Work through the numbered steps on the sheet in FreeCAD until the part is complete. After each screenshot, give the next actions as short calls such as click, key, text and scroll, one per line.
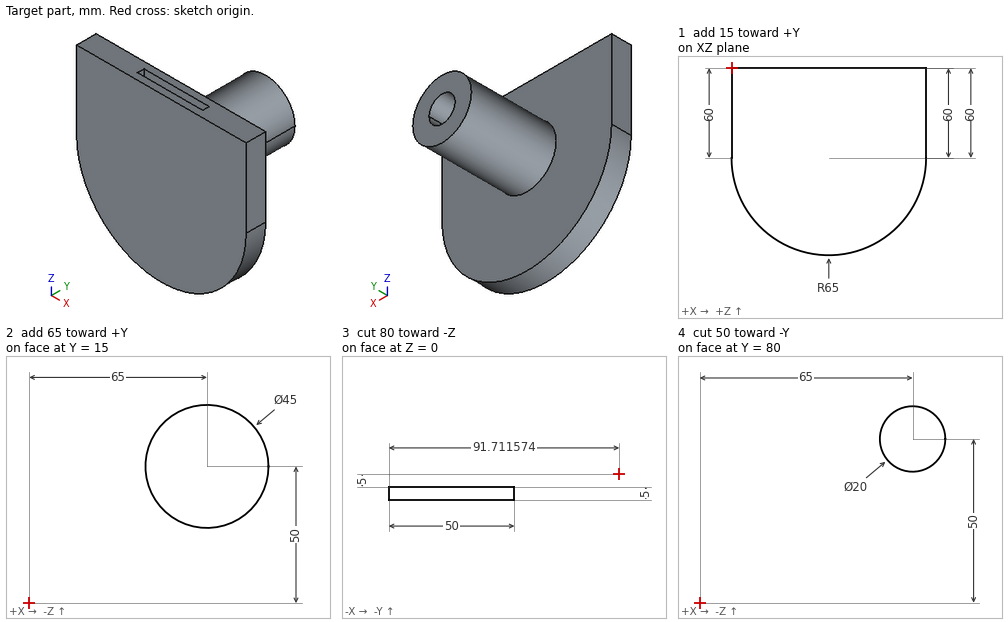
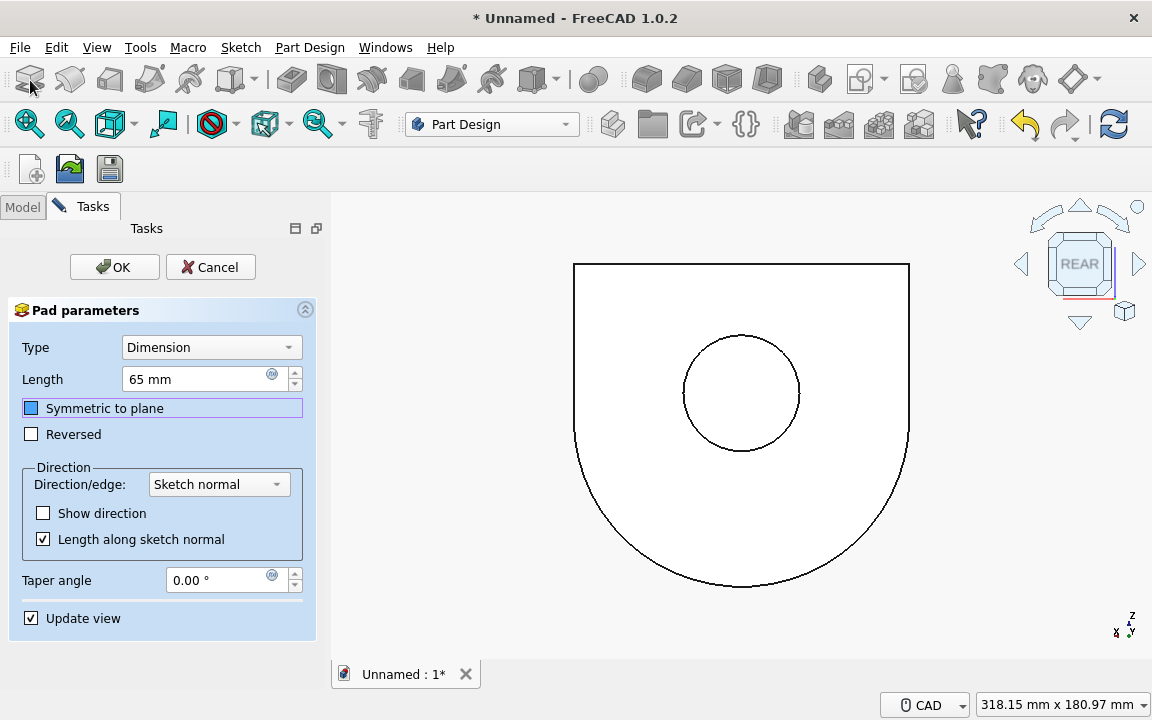
click(115, 267)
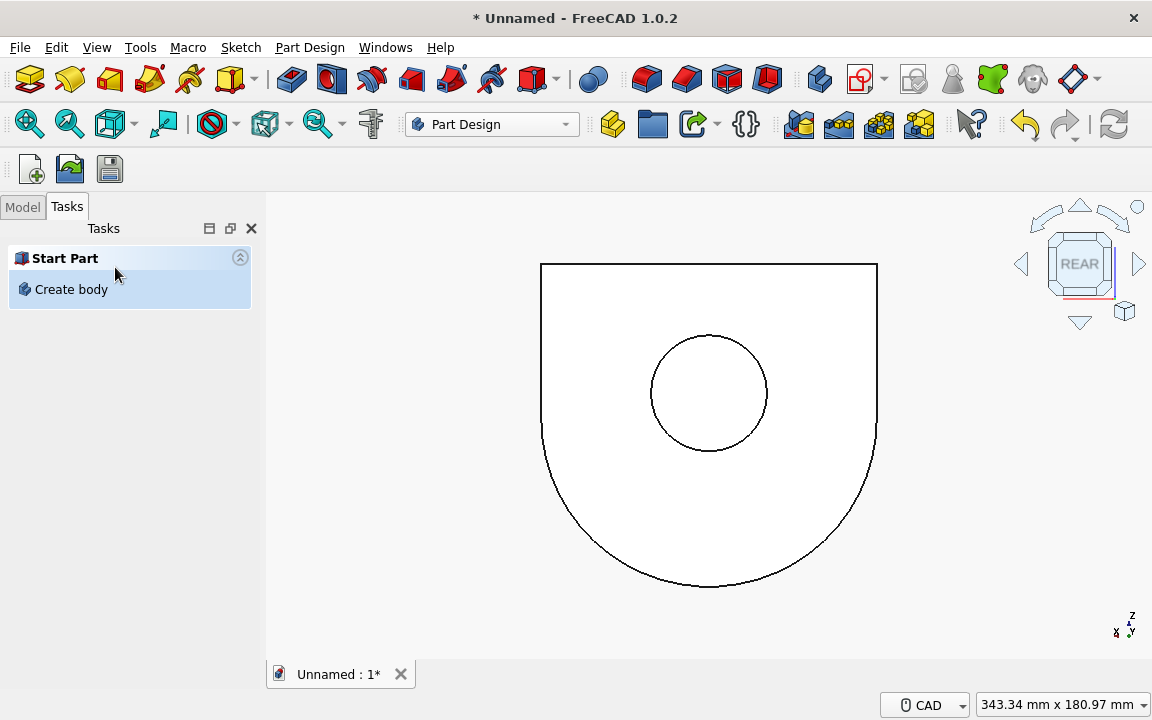
key(0)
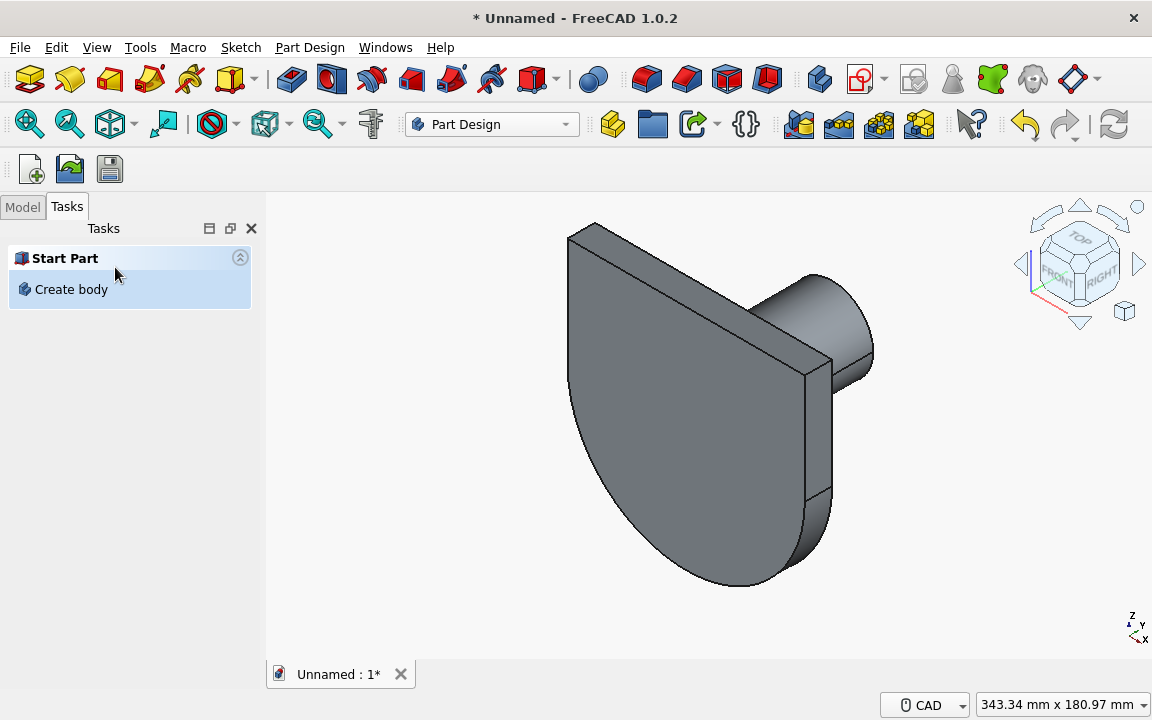
click(30, 124)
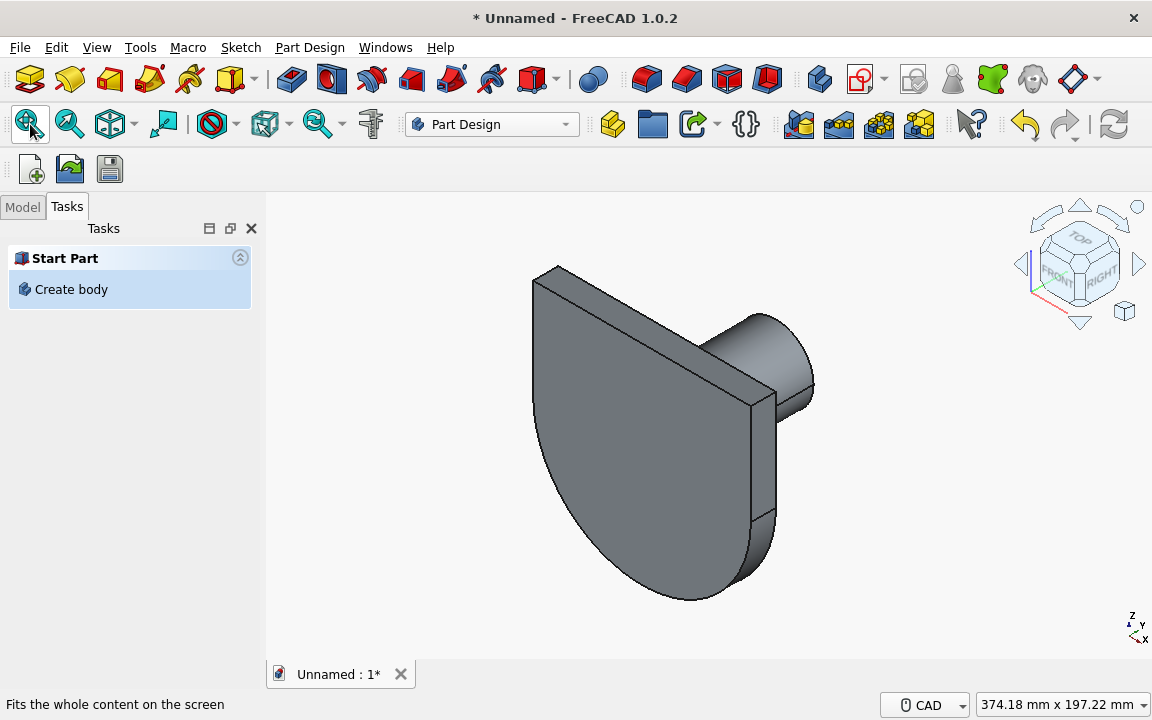
click(748, 389)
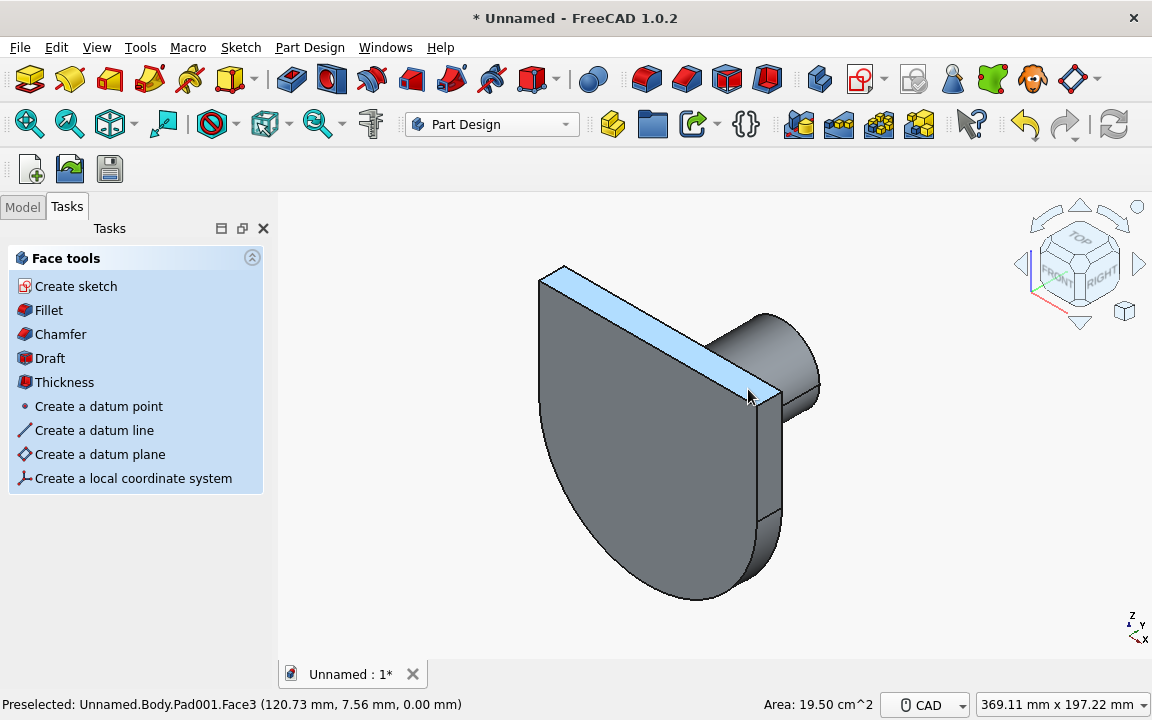
click(860, 80)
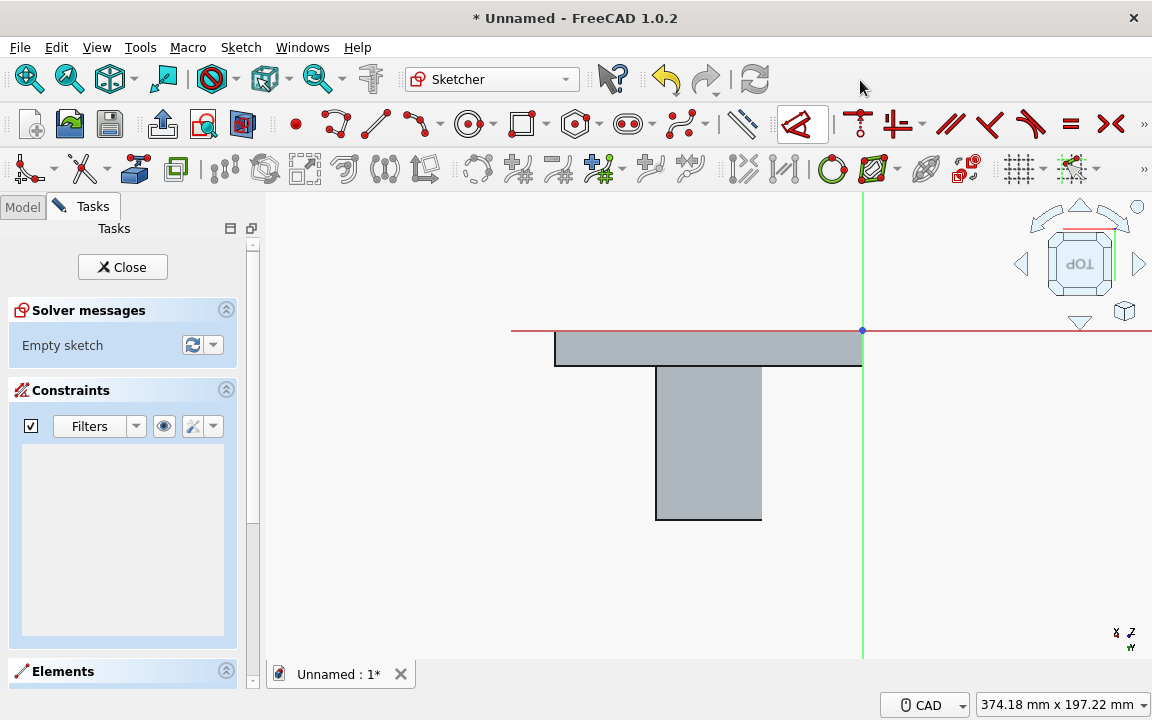
scroll(847, 275, up, 4)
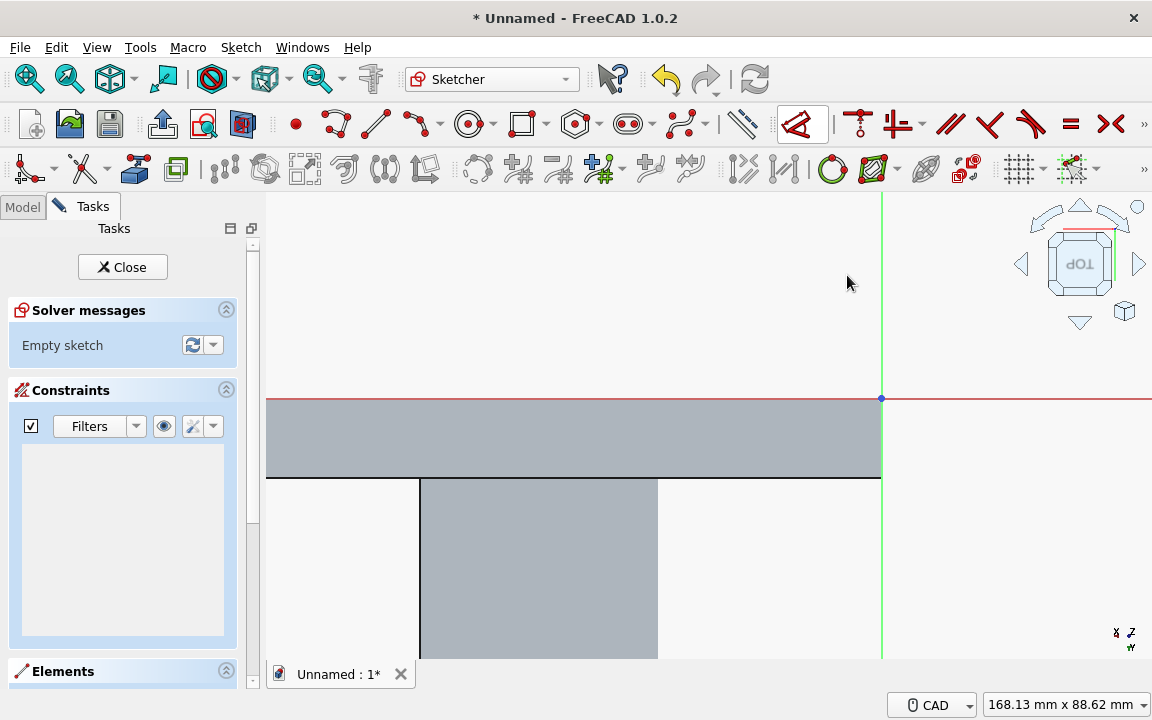
click(522, 124)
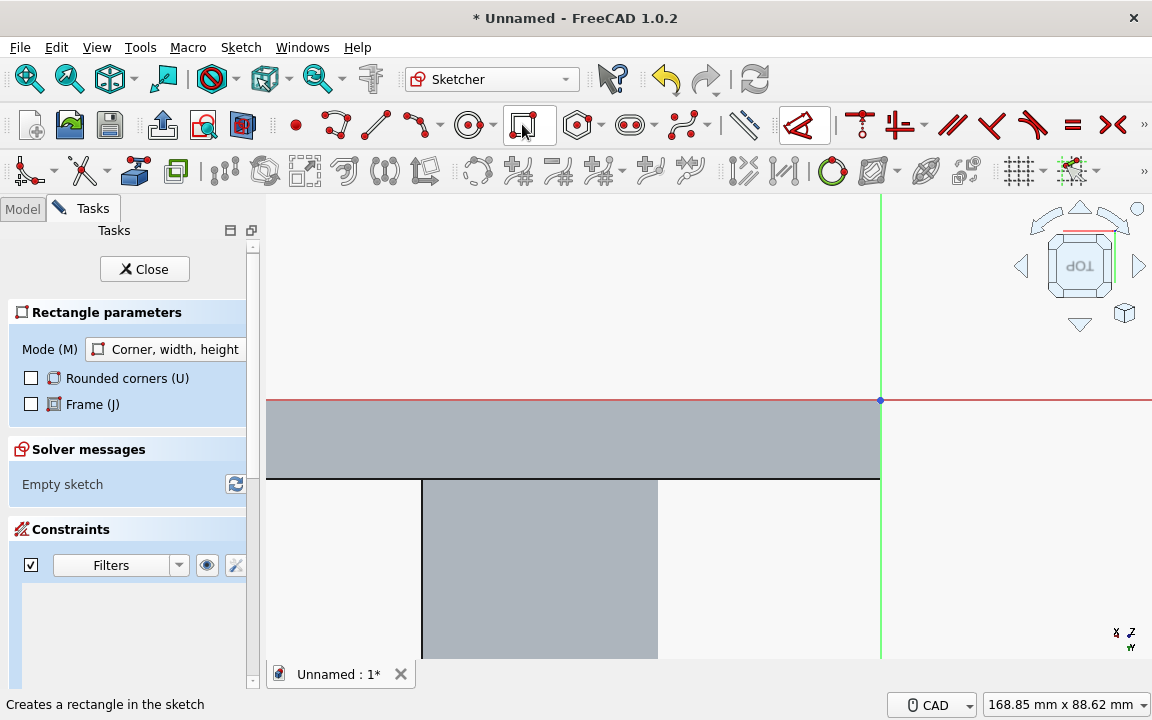
click(400, 426)
move(662, 453)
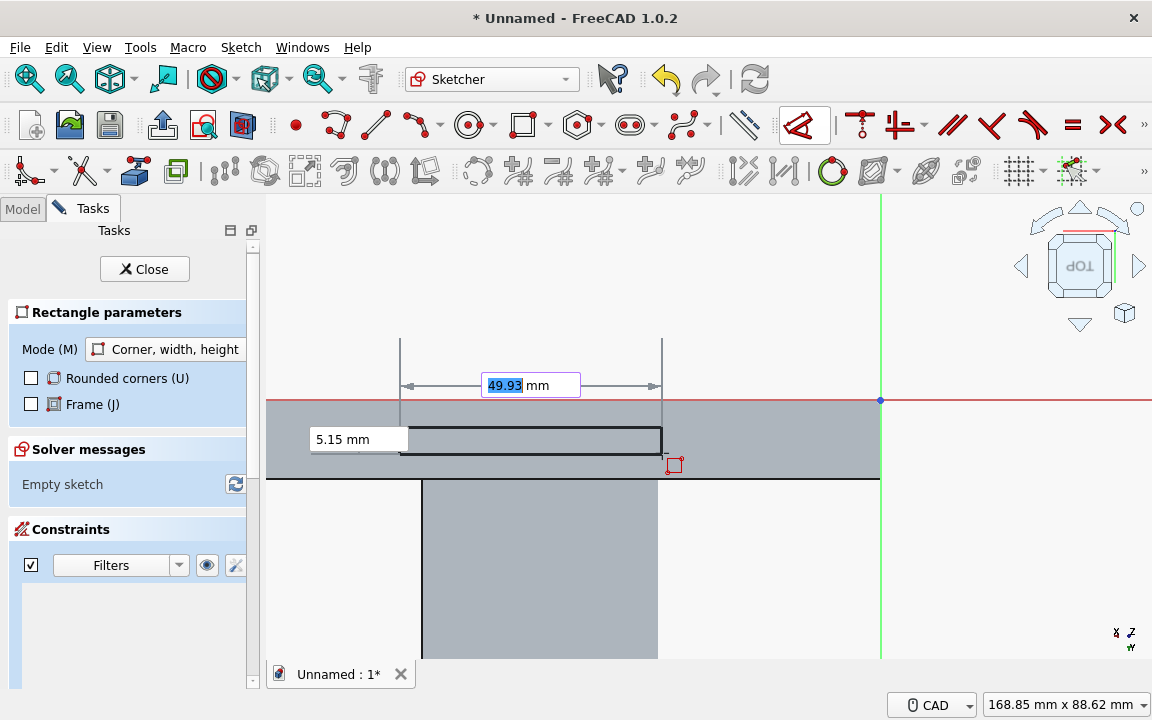
text(50)
key(Tab)
text(5)
key(Return)
key(Escape)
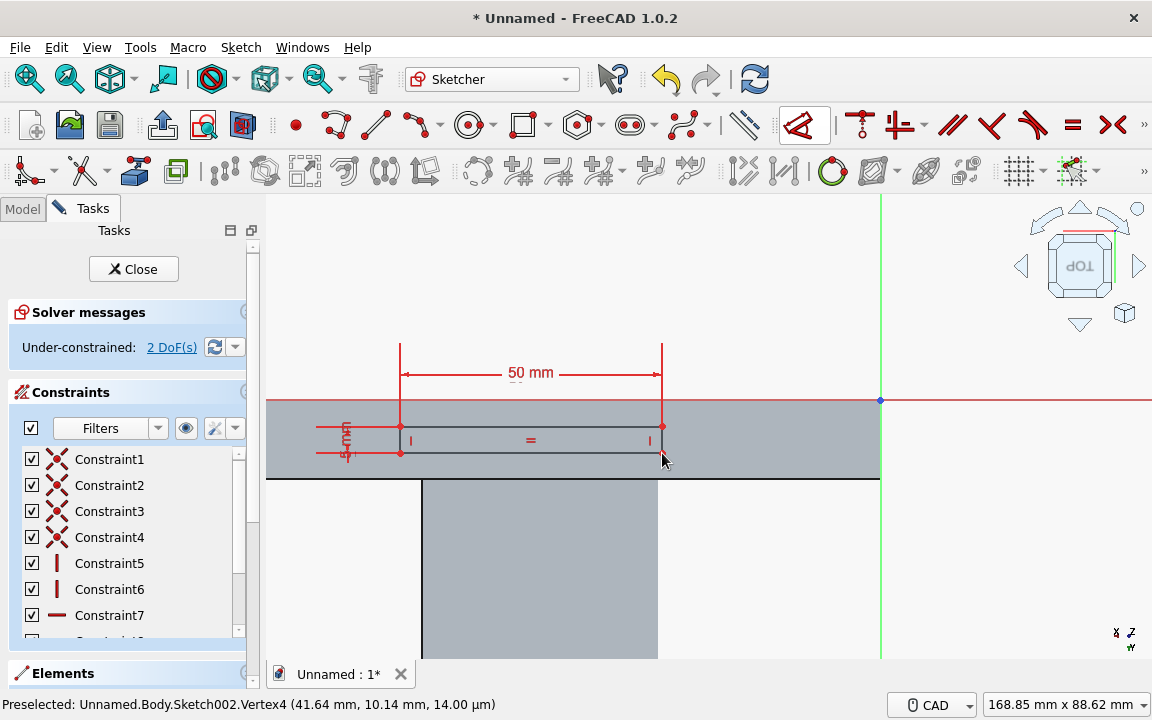
scroll(400, 427, up, 3)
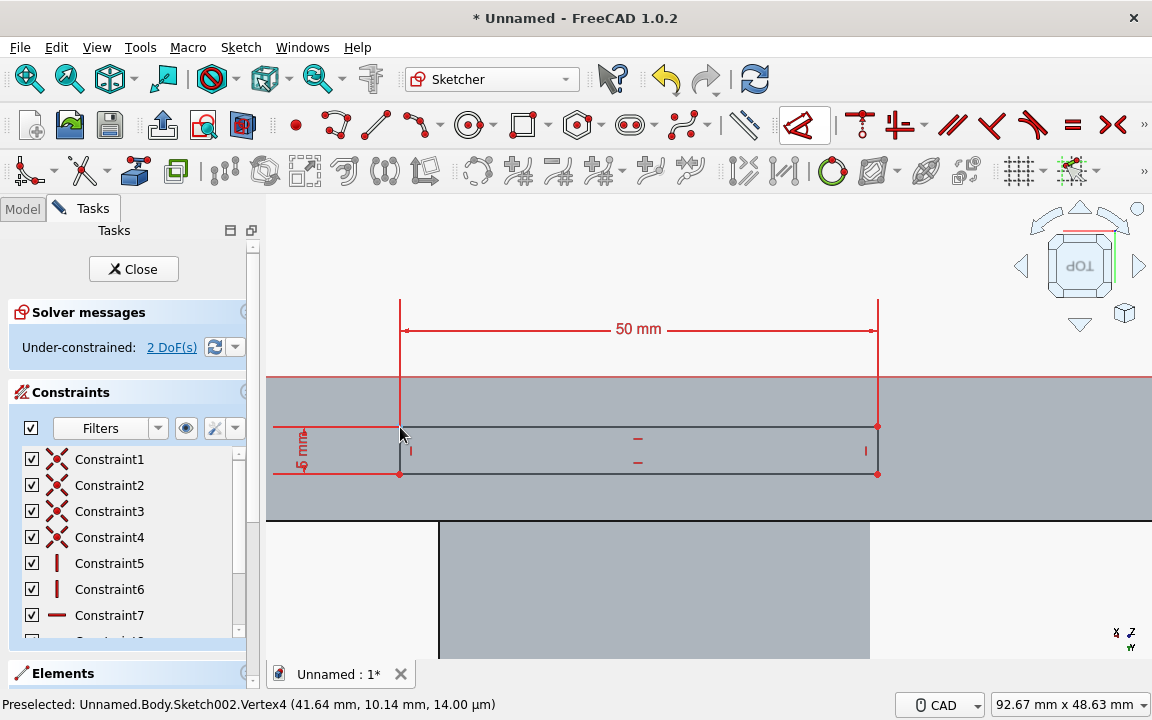
click(400, 427)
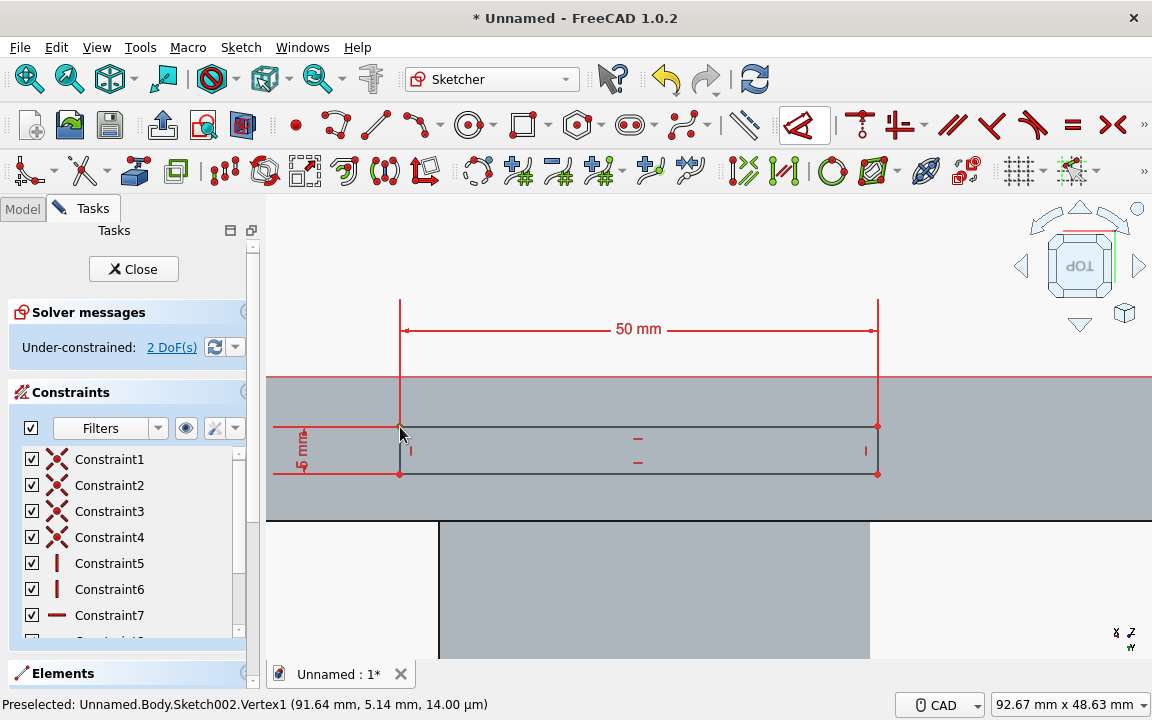
key(i)